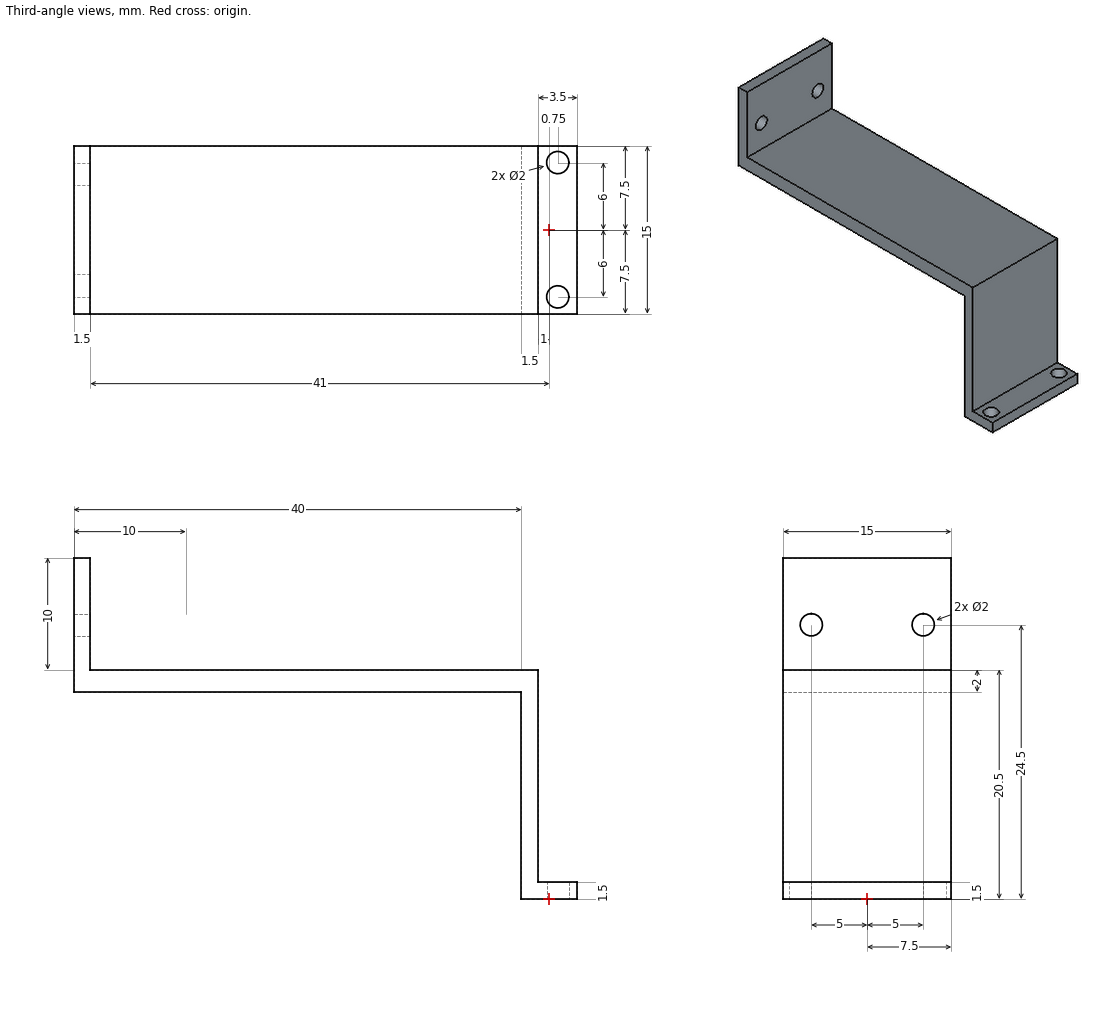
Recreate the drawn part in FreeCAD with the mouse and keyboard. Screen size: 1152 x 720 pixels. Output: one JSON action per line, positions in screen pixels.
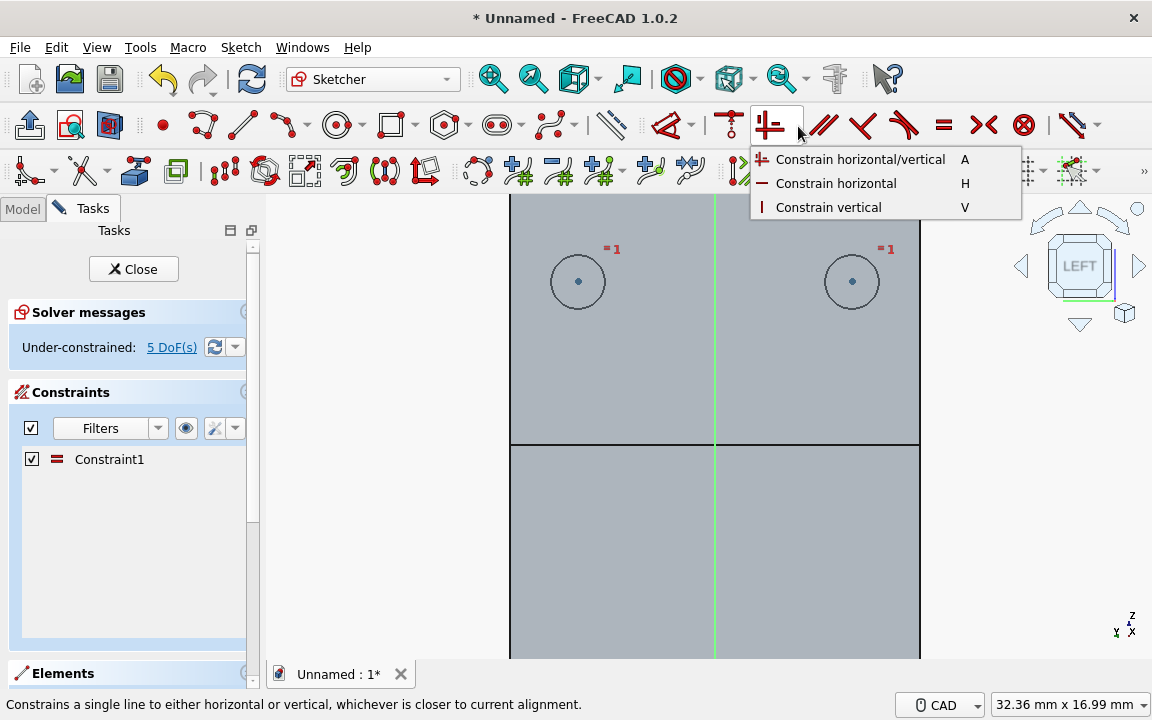
{"action": "left_click", "coordinate": [886, 183]}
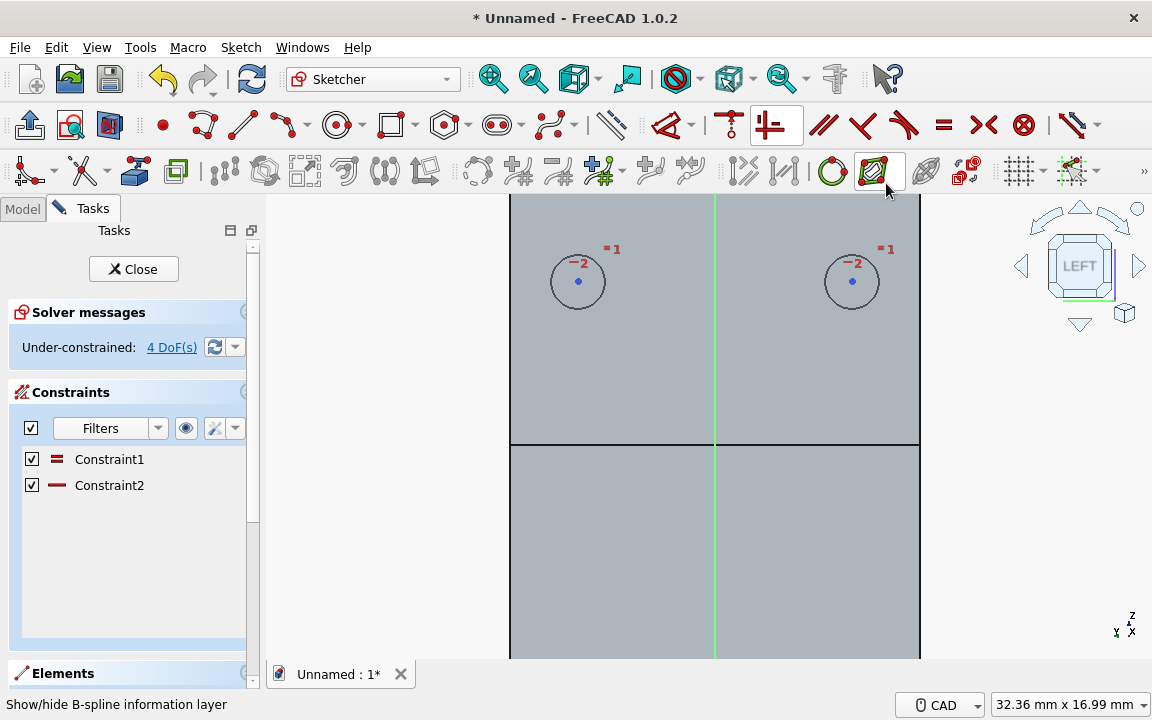
{"action": "left_click", "coordinate": [666, 126]}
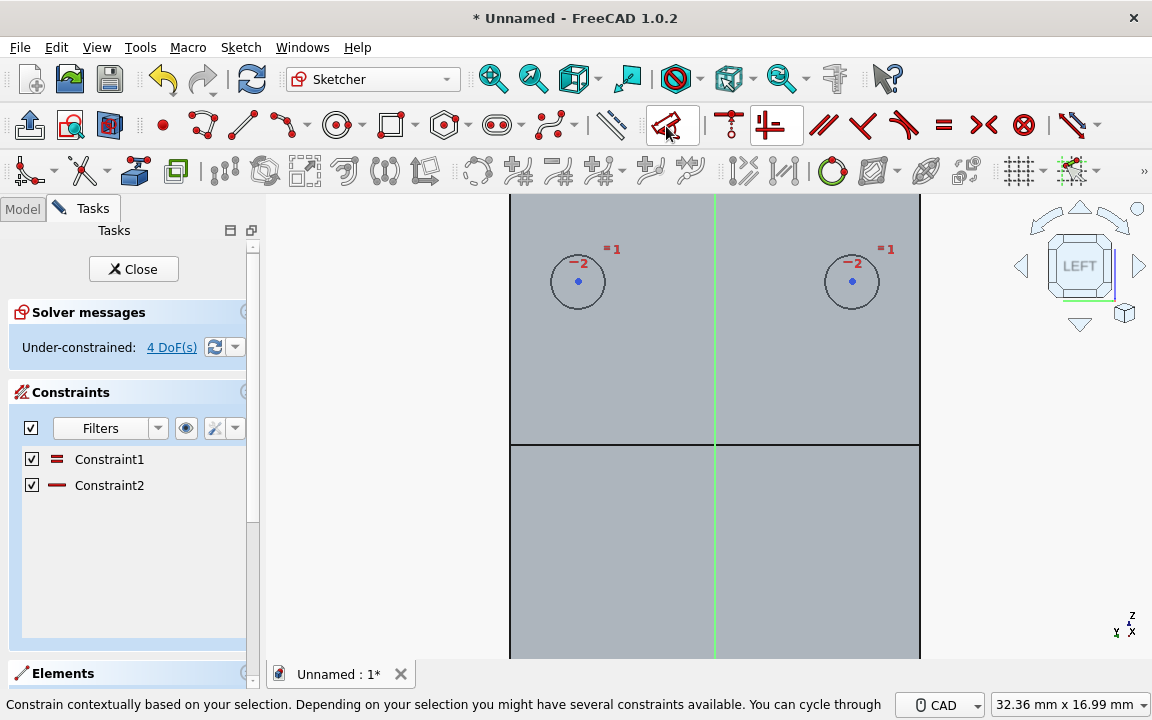
{"action": "left_click", "coordinate": [597, 263]}
{"action": "left_click", "coordinate": [620, 240]}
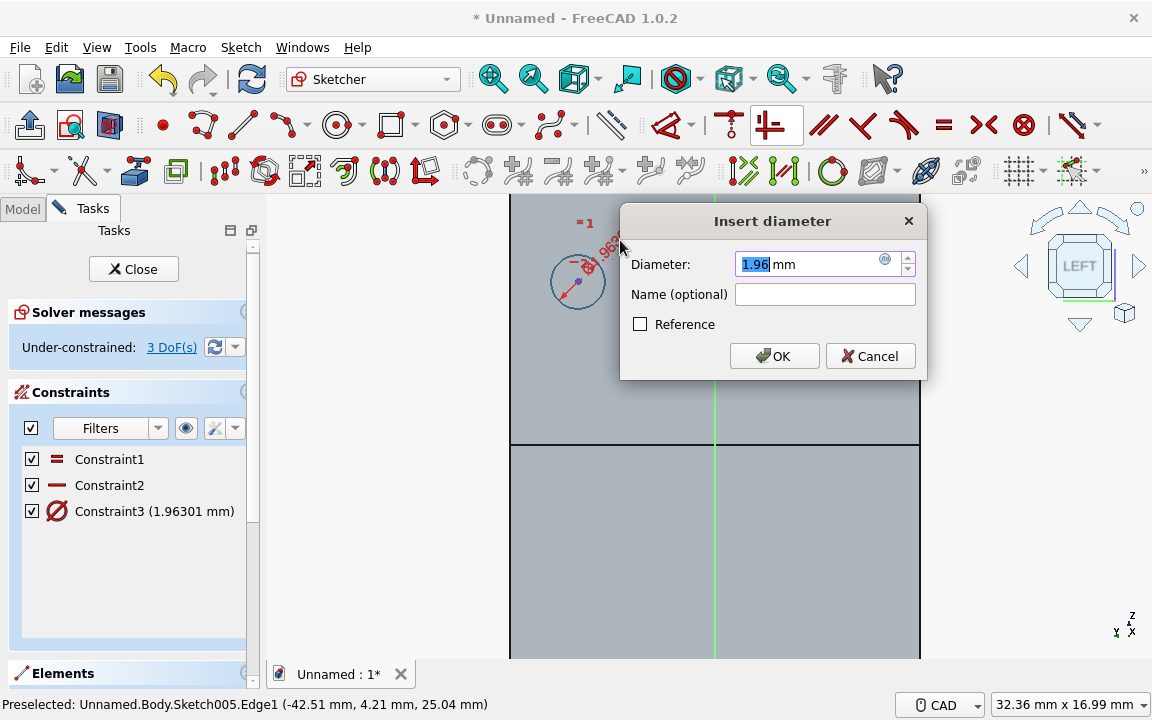
{"action": "type", "text": "2"}
{"action": "key", "text": "Return"}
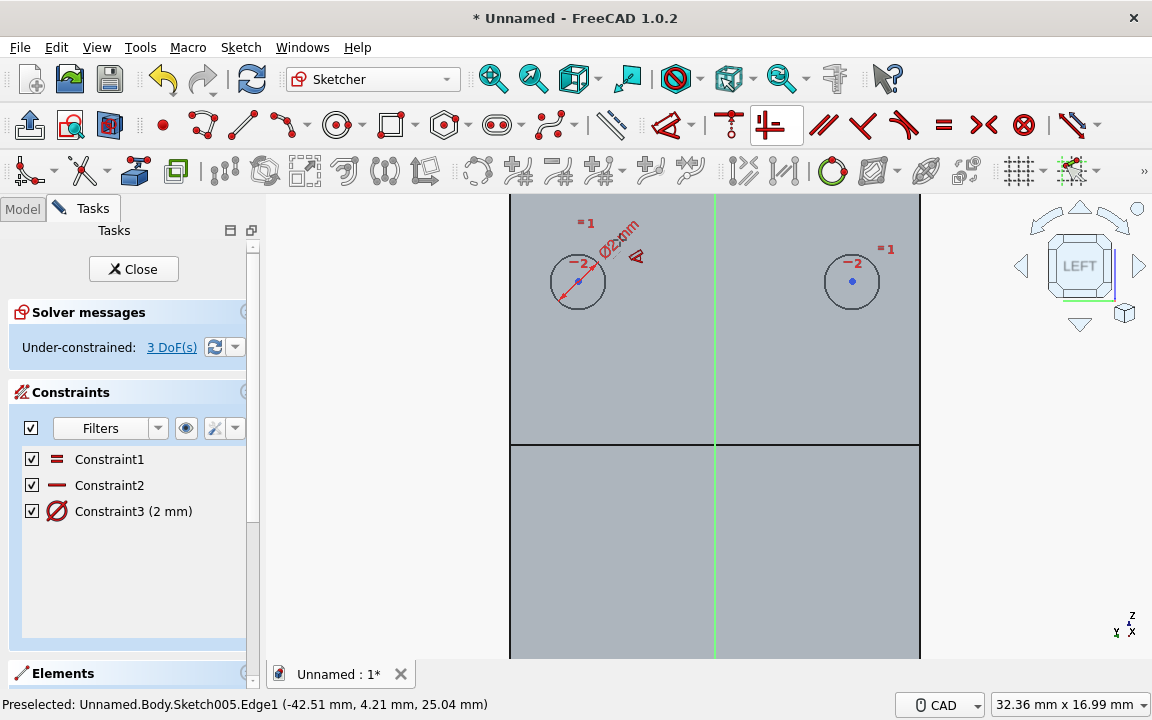
{"action": "left_click", "coordinate": [578, 282]}
{"action": "left_click", "coordinate": [694, 248]}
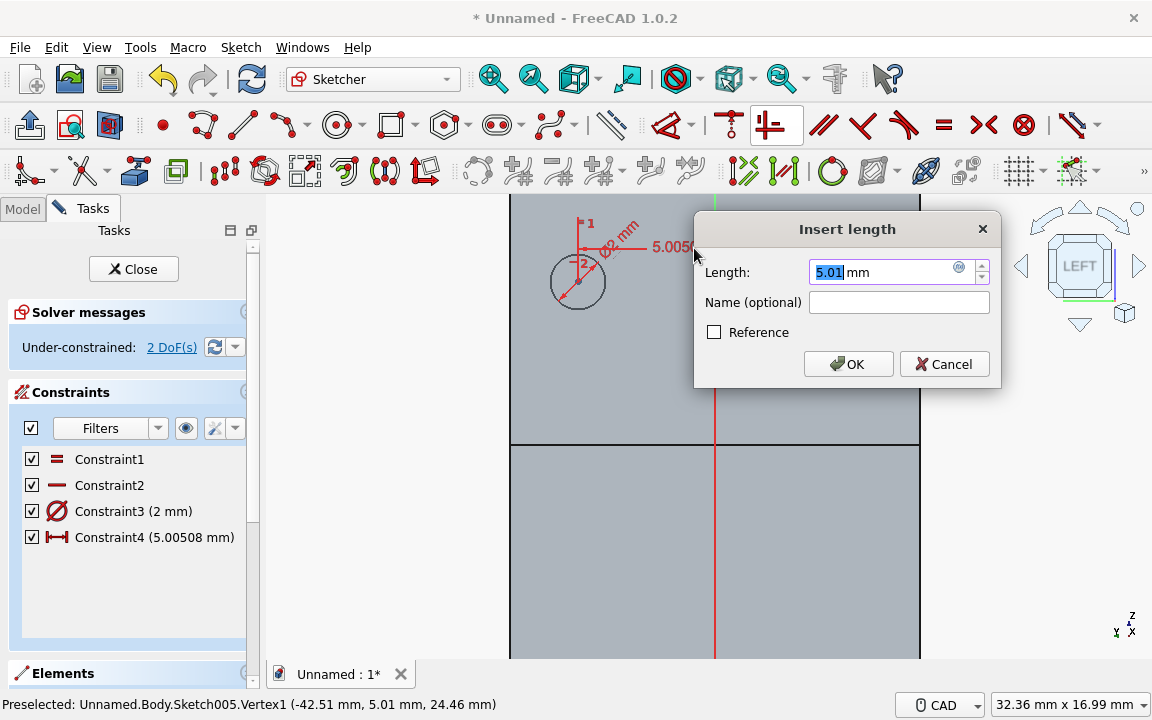
{"action": "type", "text": "5"}
{"action": "key", "text": "Return"}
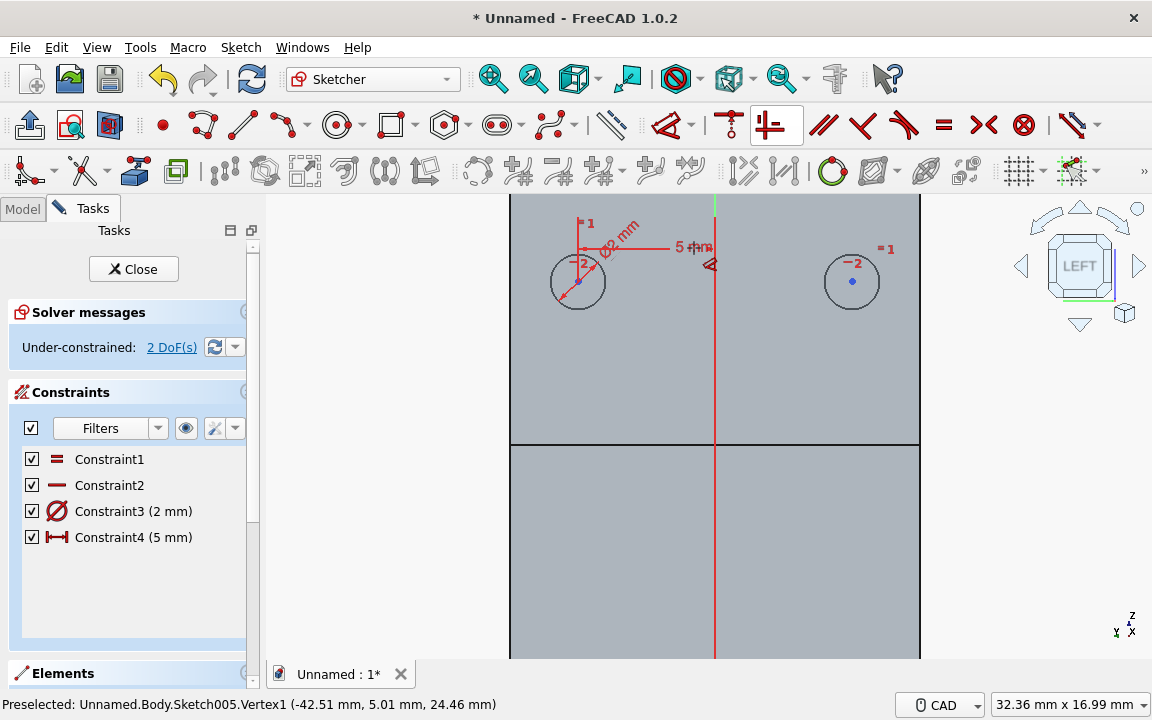
{"action": "left_click", "coordinate": [852, 282]}
{"action": "left_click", "coordinate": [784, 248]}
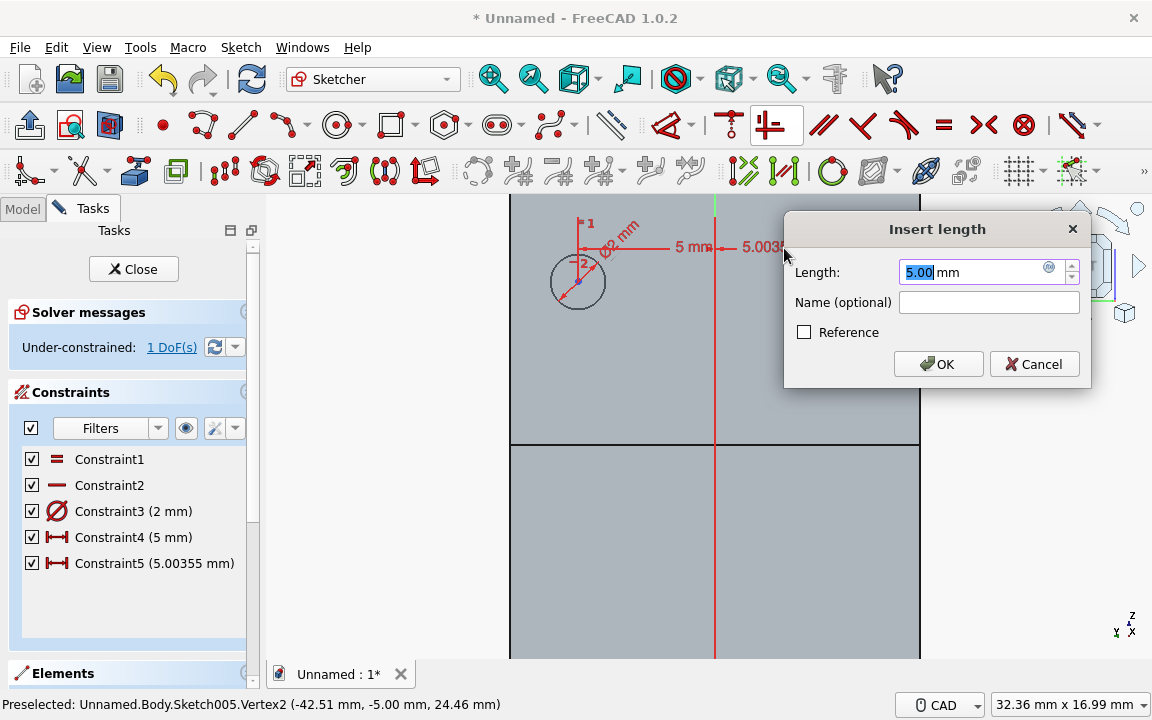
{"action": "type", "text": "5"}
{"action": "key", "text": "Return"}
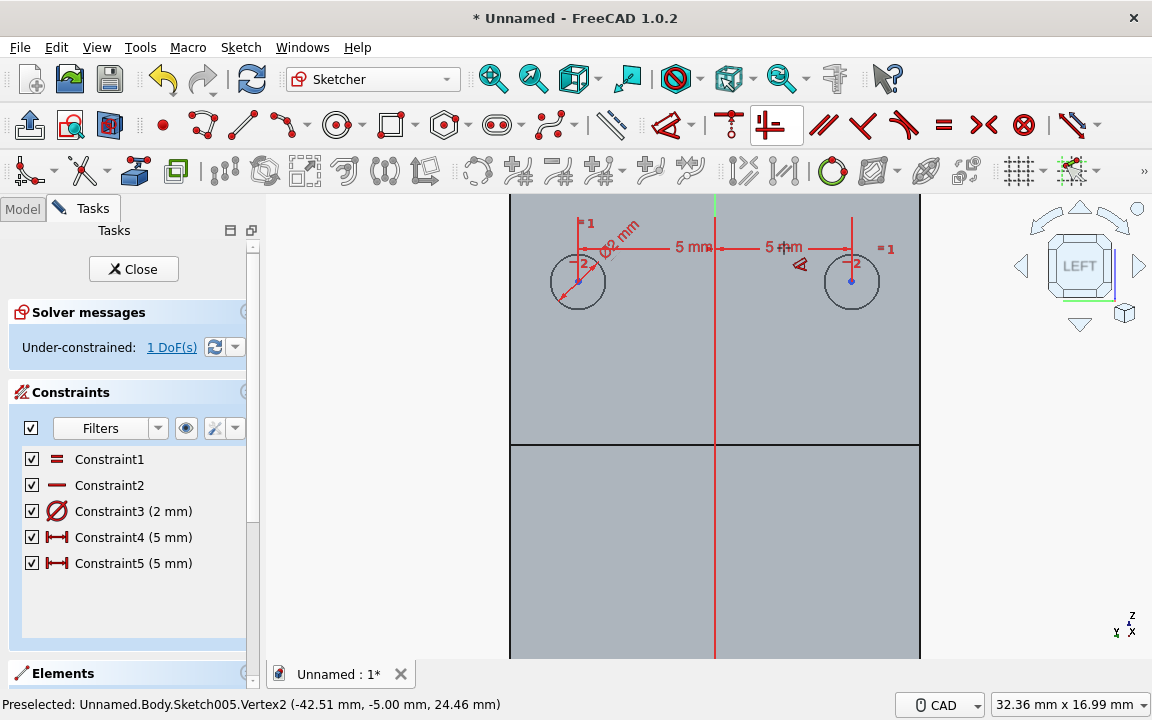
{"action": "left_click", "coordinate": [578, 282]}
{"action": "left_click", "coordinate": [544, 457]}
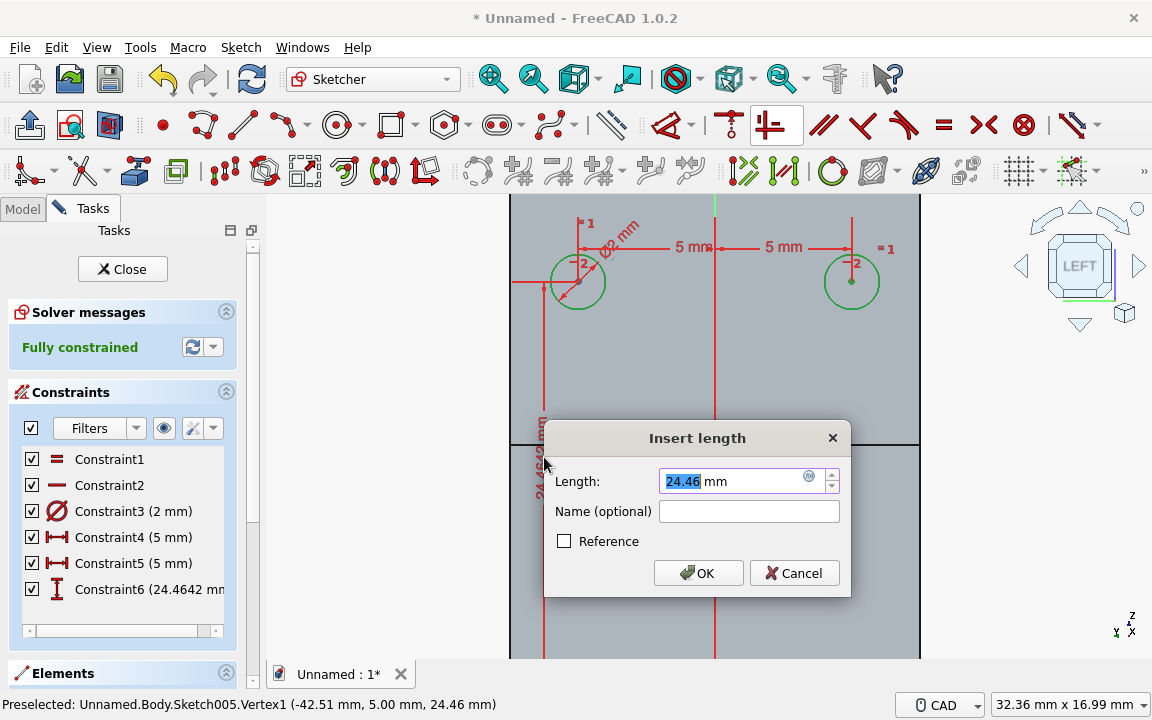
{"action": "type", "text": "24.5"}
{"action": "key", "text": "Return"}
{"action": "key", "text": "Escape"}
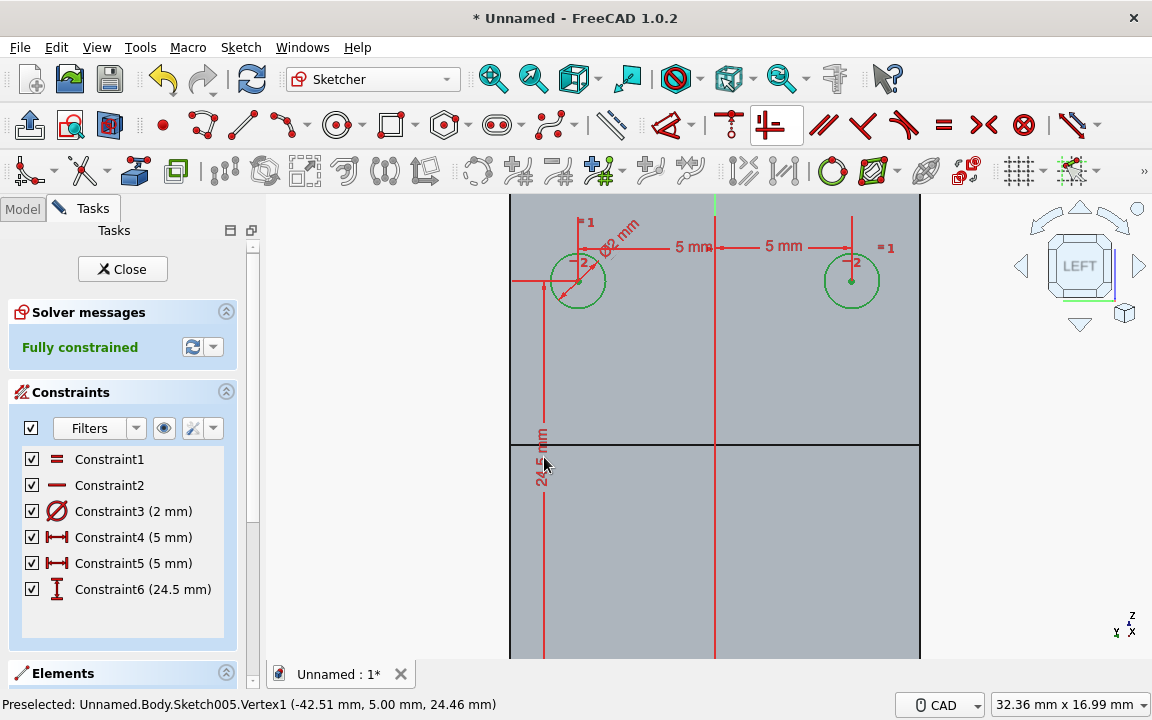
{"action": "left_click", "coordinate": [123, 269]}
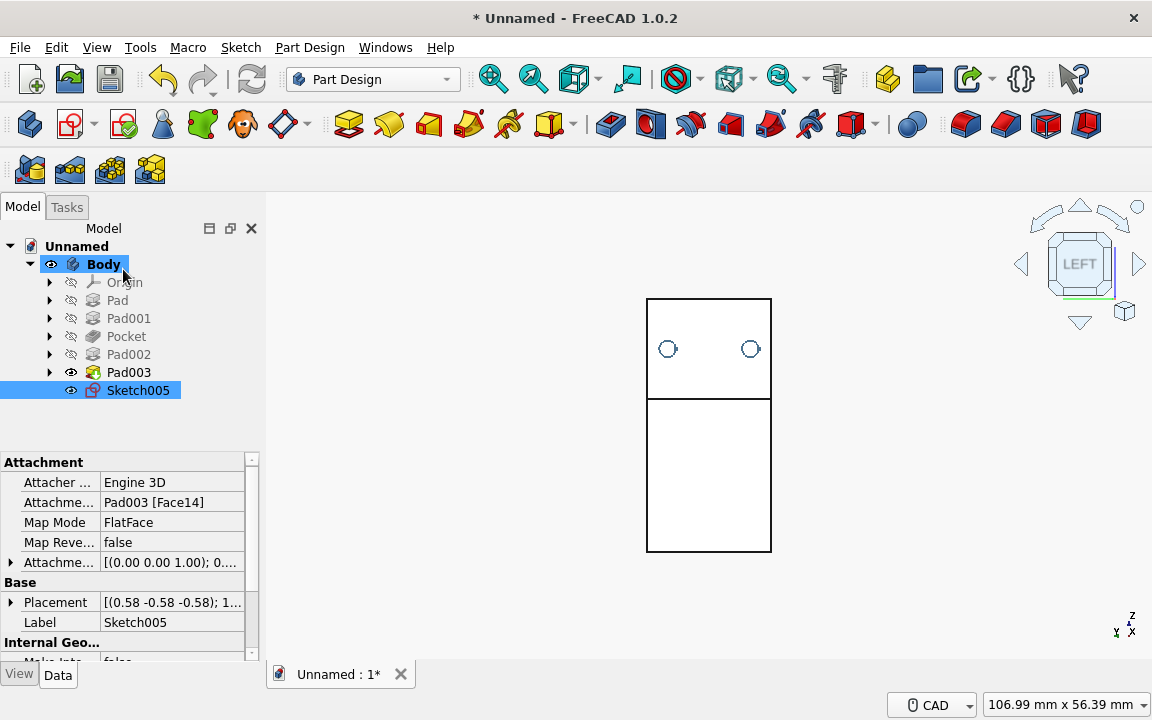
{"action": "left_click", "coordinate": [612, 124]}